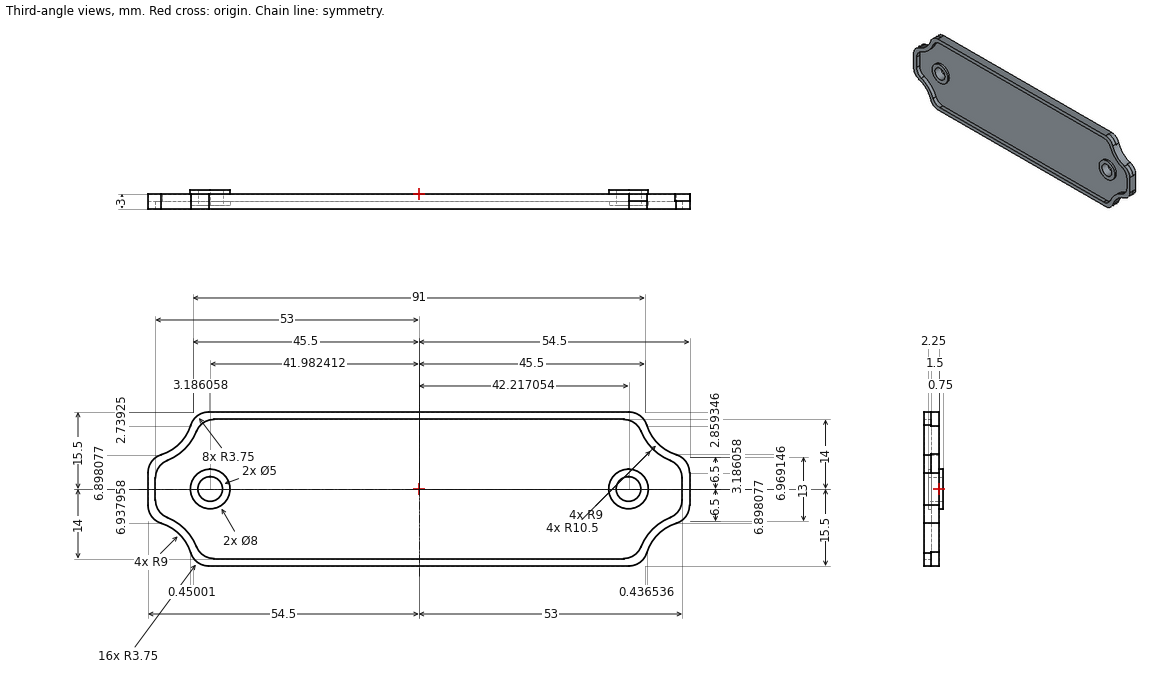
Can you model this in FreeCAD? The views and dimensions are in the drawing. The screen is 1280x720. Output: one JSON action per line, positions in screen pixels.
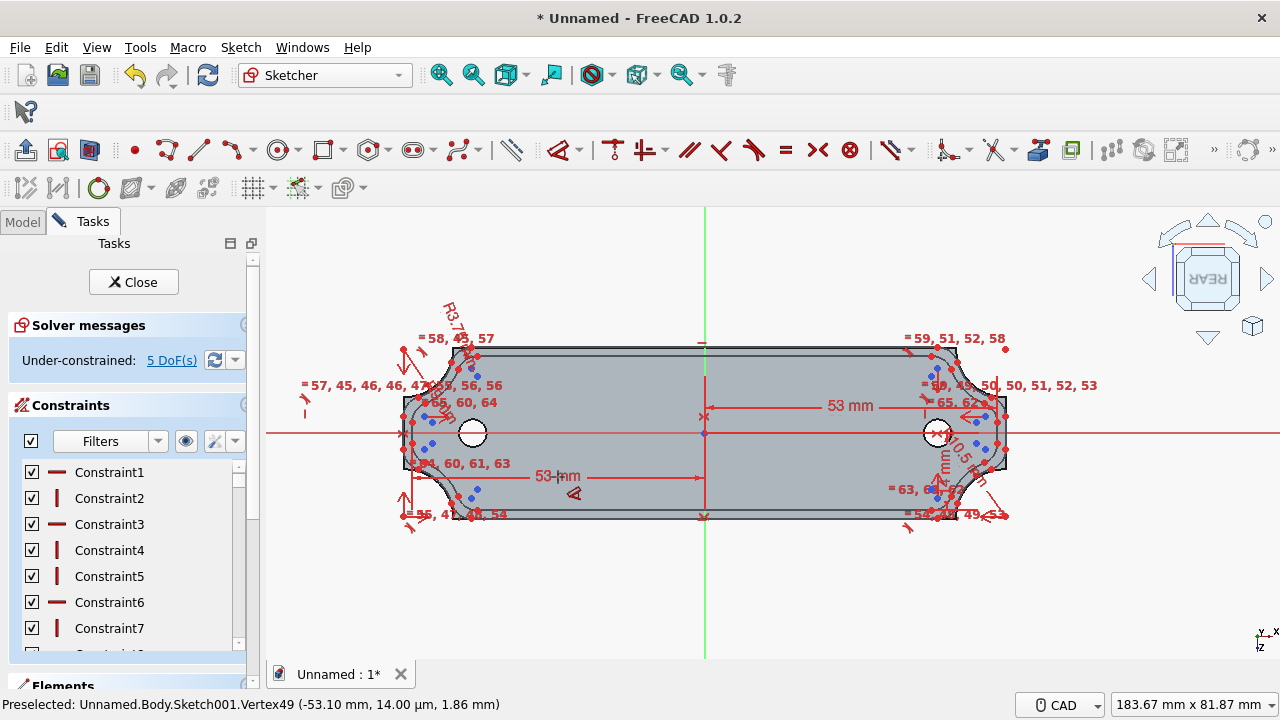
{"action": "left_click", "coordinate": [478, 356]}
{"action": "left_click", "coordinate": [739, 395]}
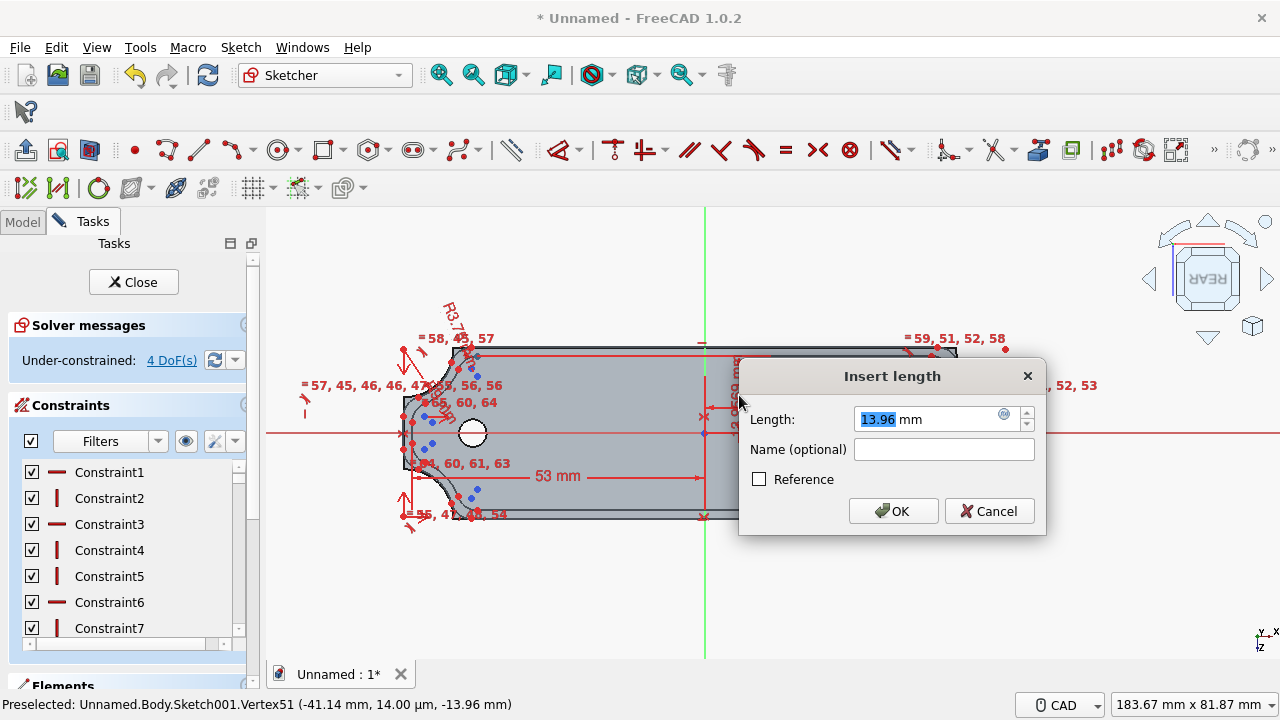
{"action": "type", "text": "14"}
{"action": "key", "text": "Return"}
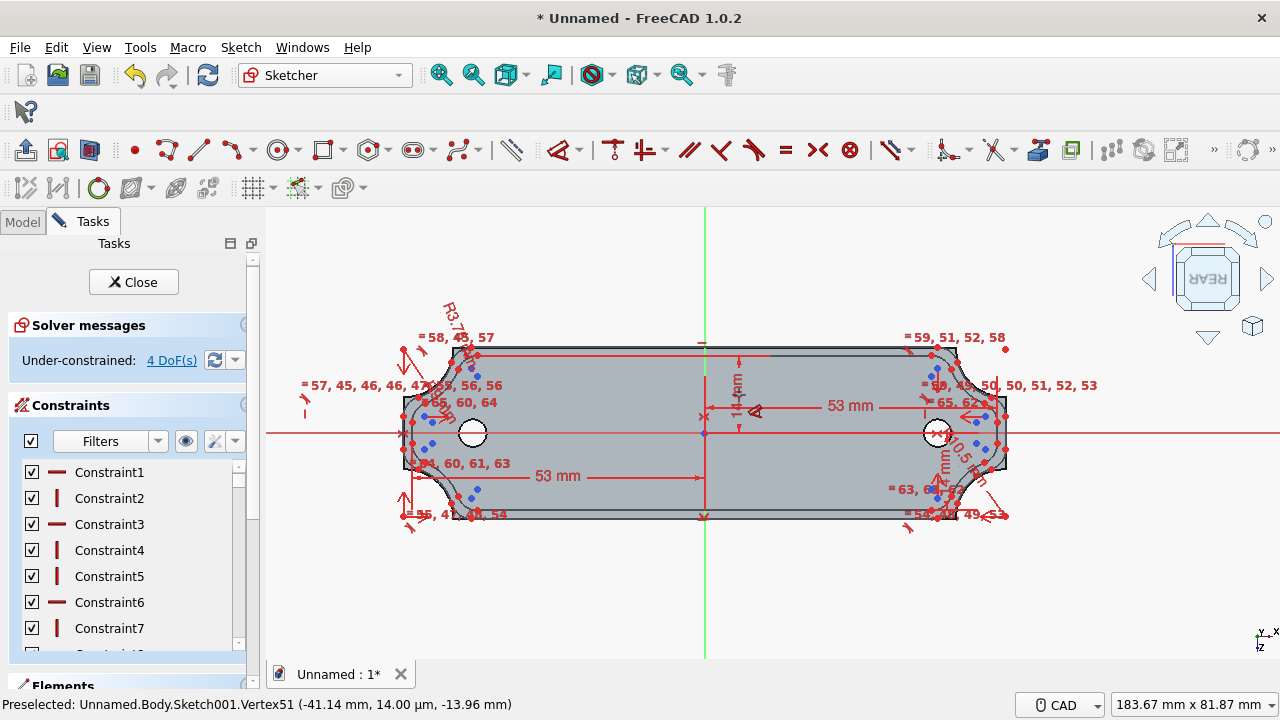
{"action": "left_click", "coordinate": [938, 347]}
{"action": "left_click", "coordinate": [972, 360]}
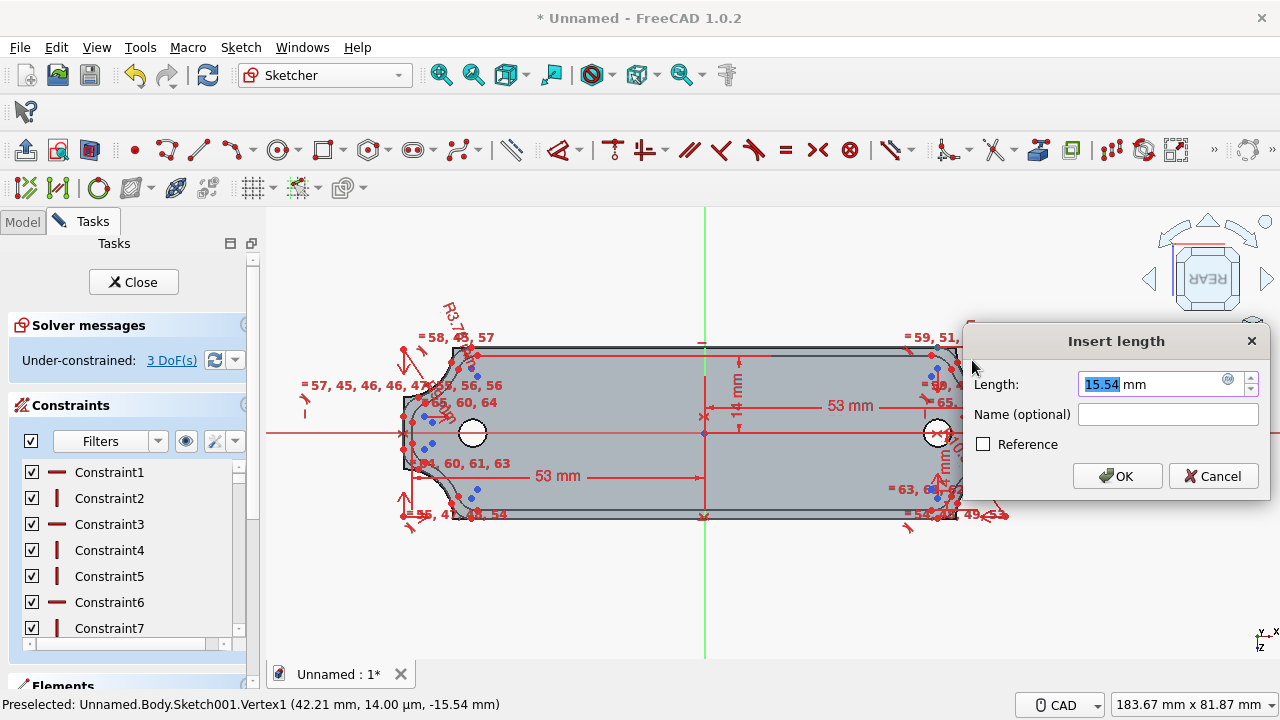
{"action": "type", "text": "15.5"}
{"action": "key", "text": "Return"}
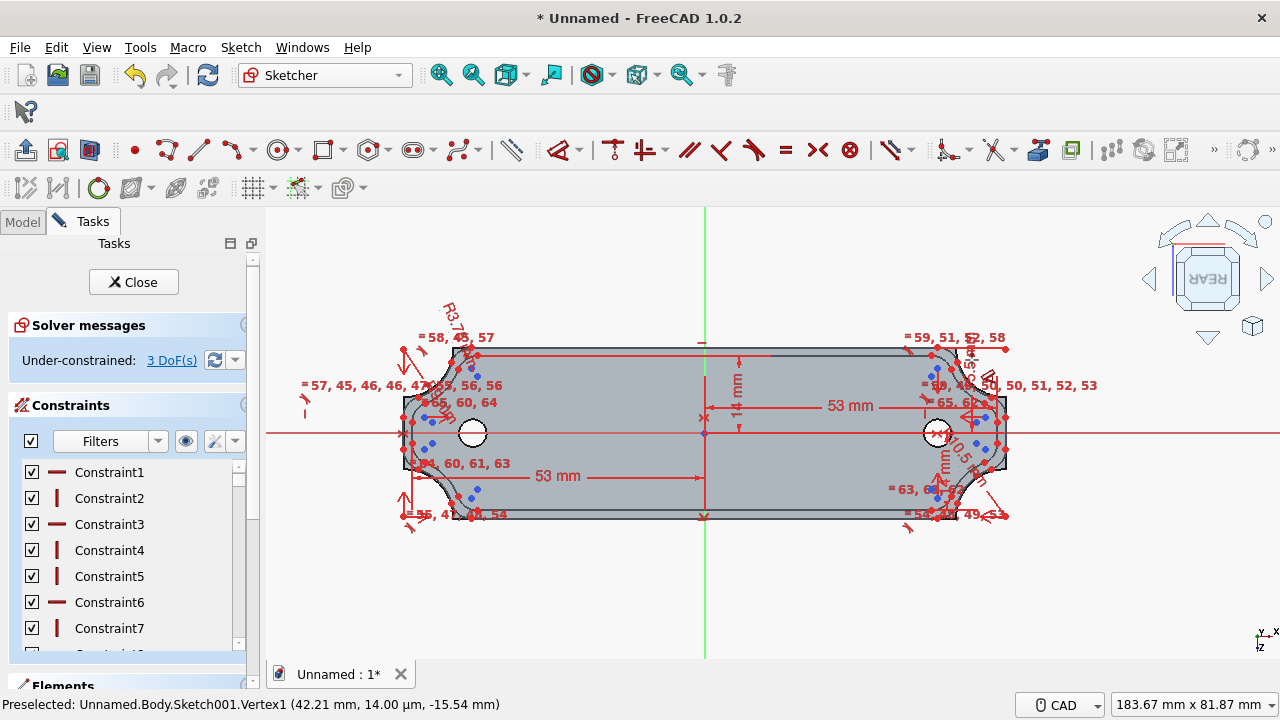
{"action": "left_click", "coordinate": [403, 417]}
{"action": "left_click", "coordinate": [554, 383]}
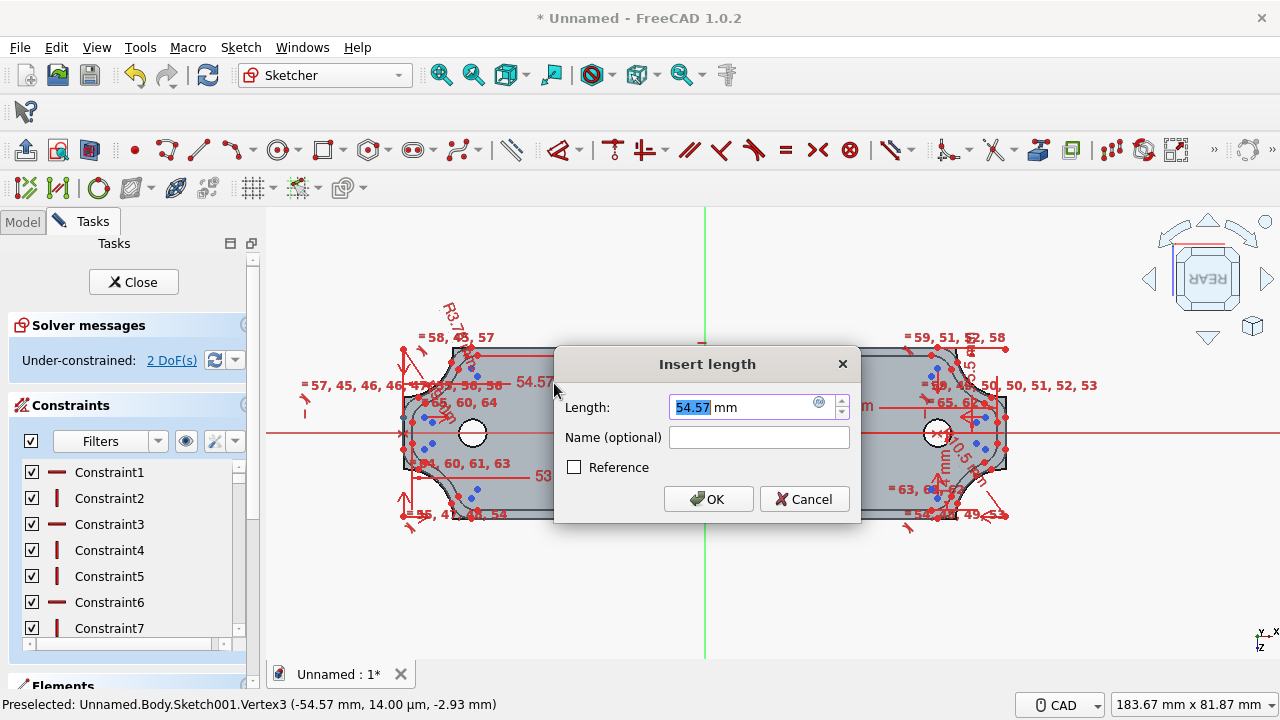
{"action": "type", "text": "54.5"}
{"action": "key", "text": "Return"}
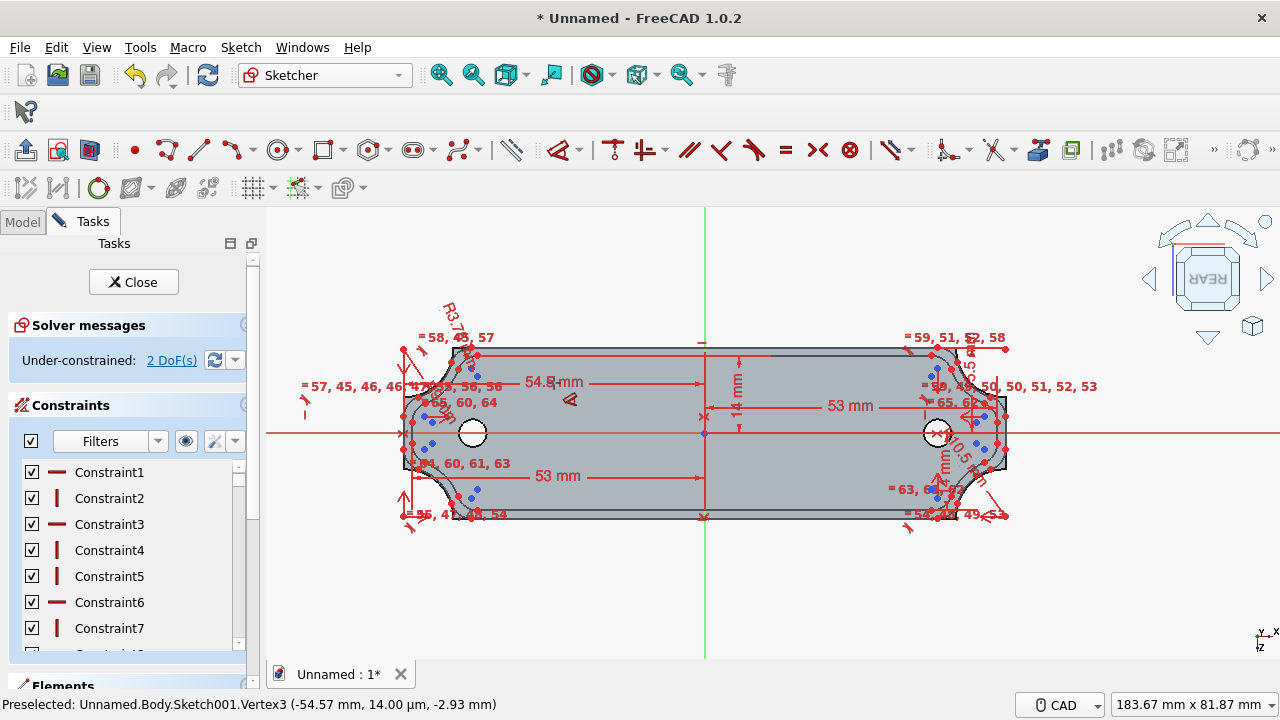
{"action": "left_click", "coordinate": [404, 350]}
{"action": "left_click", "coordinate": [554, 316]}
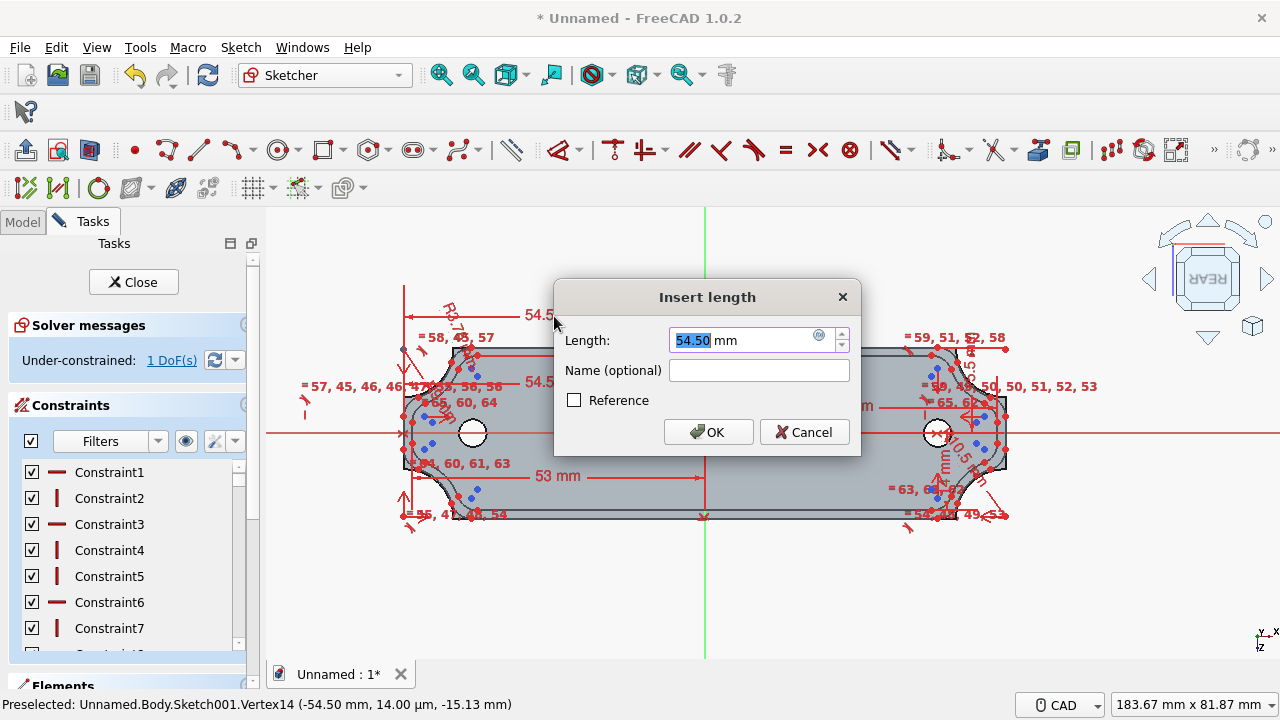
{"action": "type", "text": "54.5"}
{"action": "key", "text": "Return"}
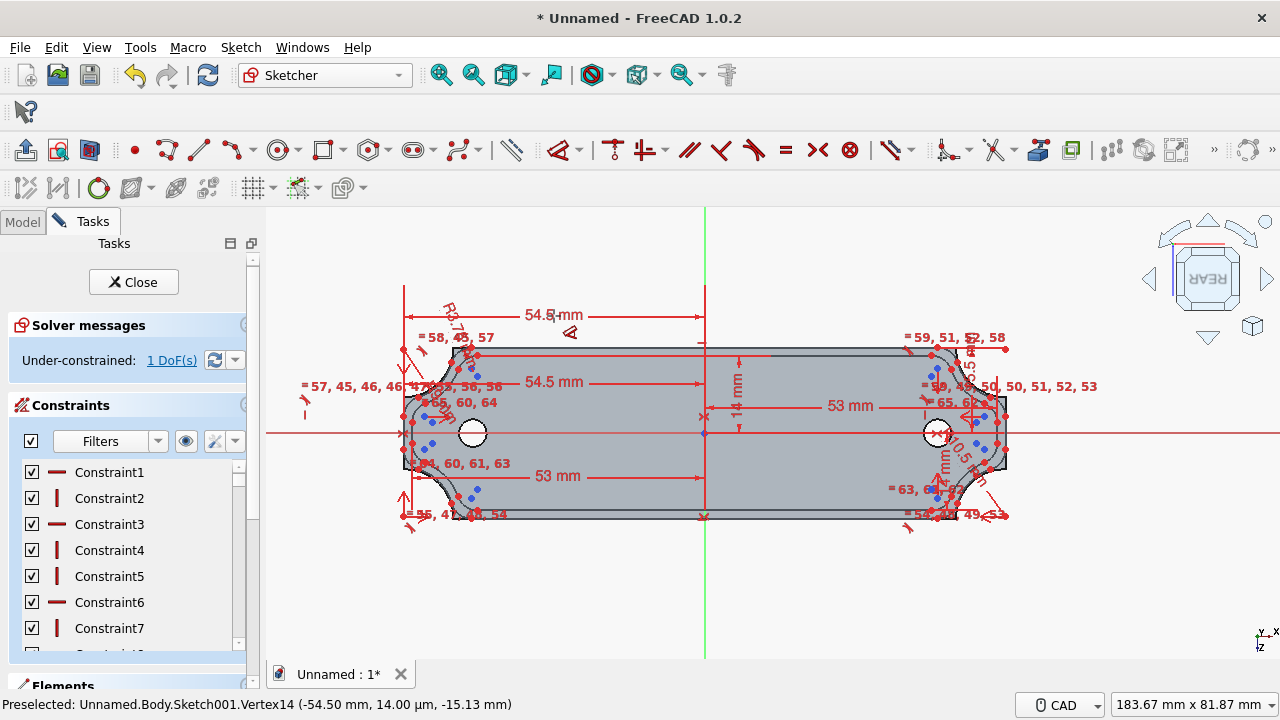
{"action": "left_click", "coordinate": [404, 350]}
{"action": "left_click", "coordinate": [370, 391]}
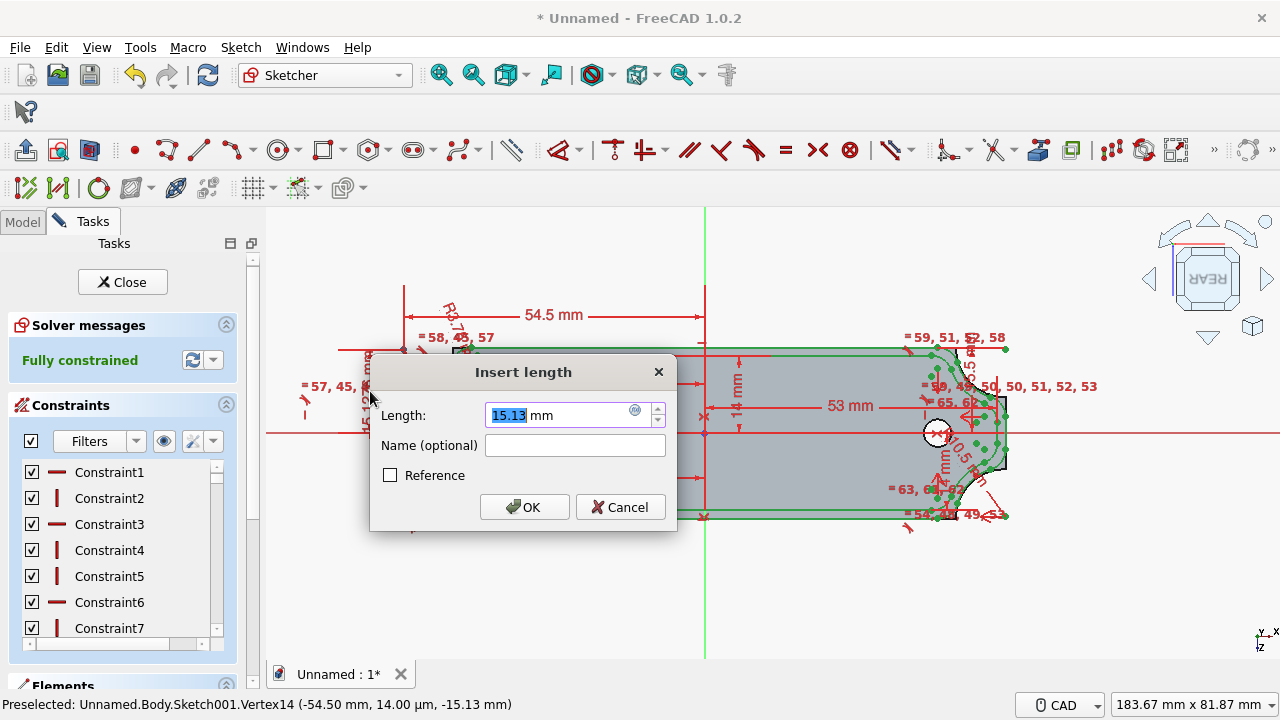
{"action": "type", "text": "15.5"}
{"action": "key", "text": "Return"}
{"action": "key", "text": "Escape"}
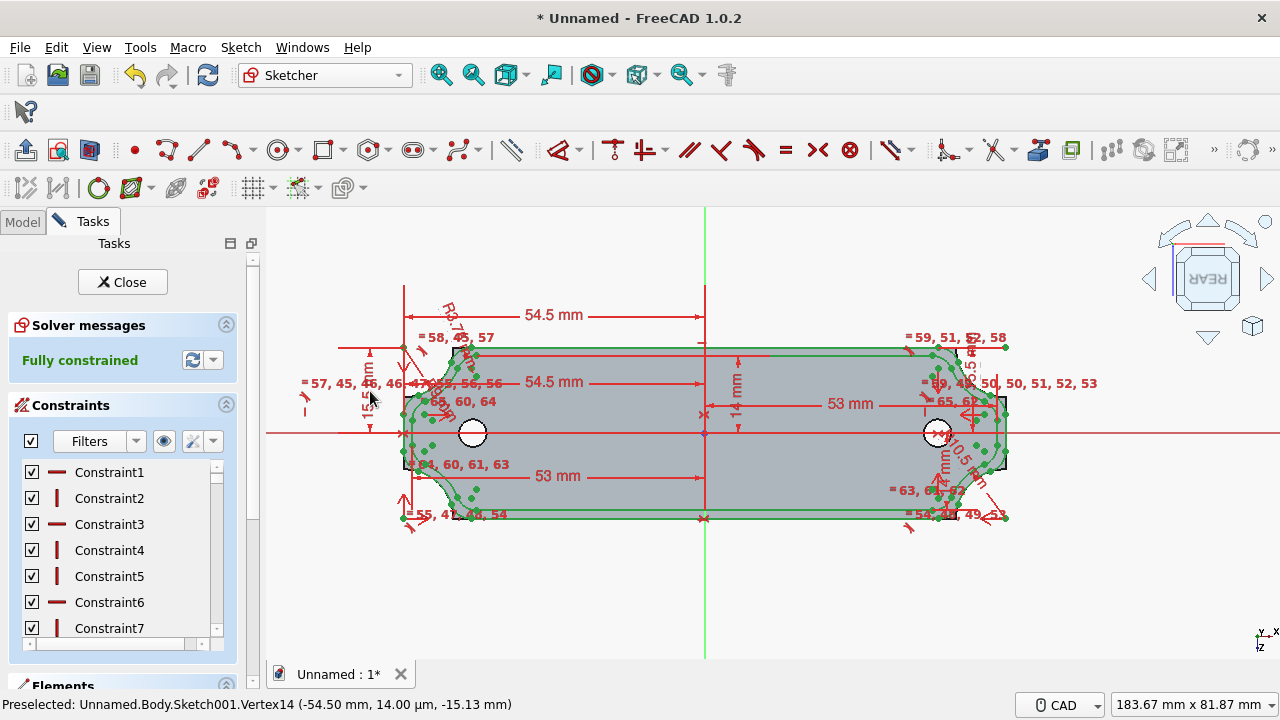
{"action": "left_click", "coordinate": [123, 282]}